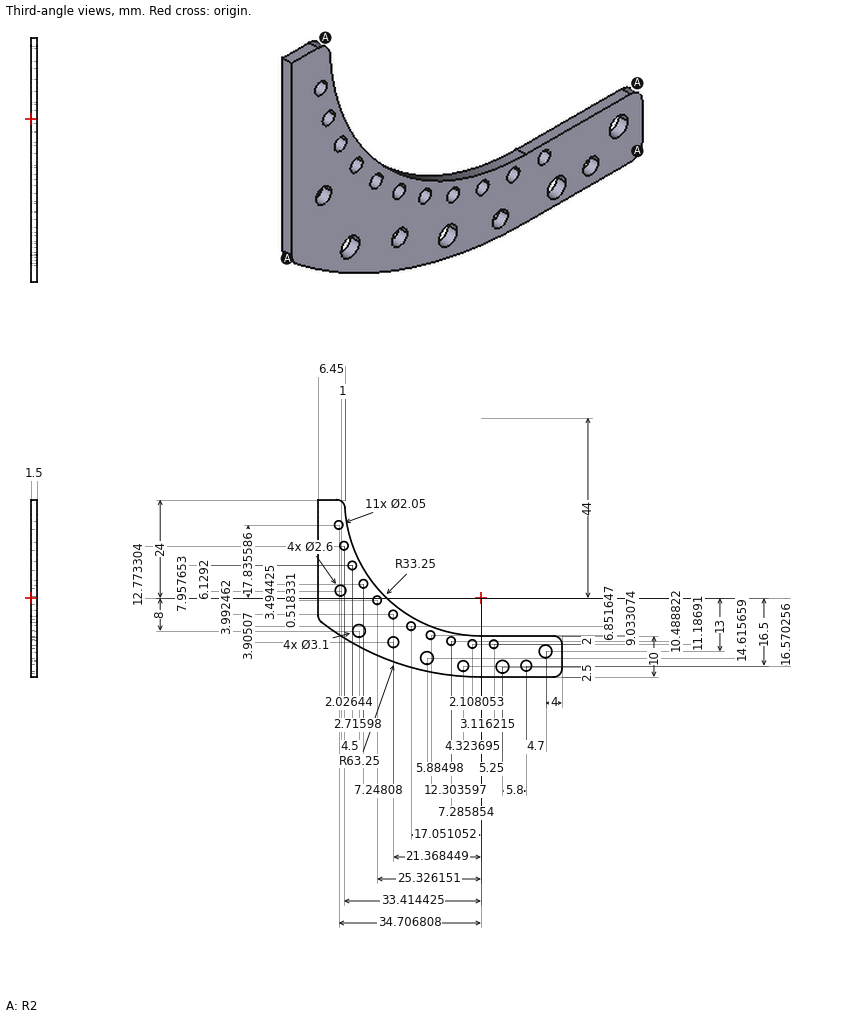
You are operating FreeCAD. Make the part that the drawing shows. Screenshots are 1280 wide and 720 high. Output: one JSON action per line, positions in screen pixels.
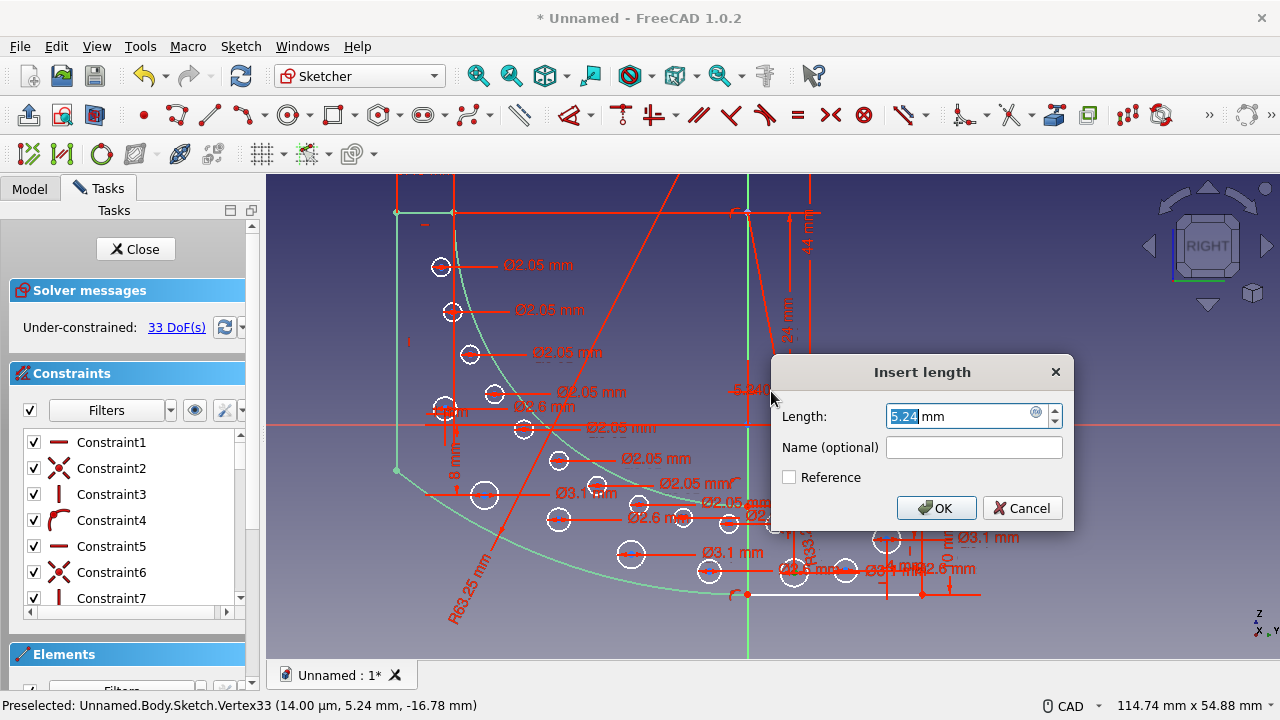
{"action": "type", "text": "5.25"}
{"action": "key", "text": "Return"}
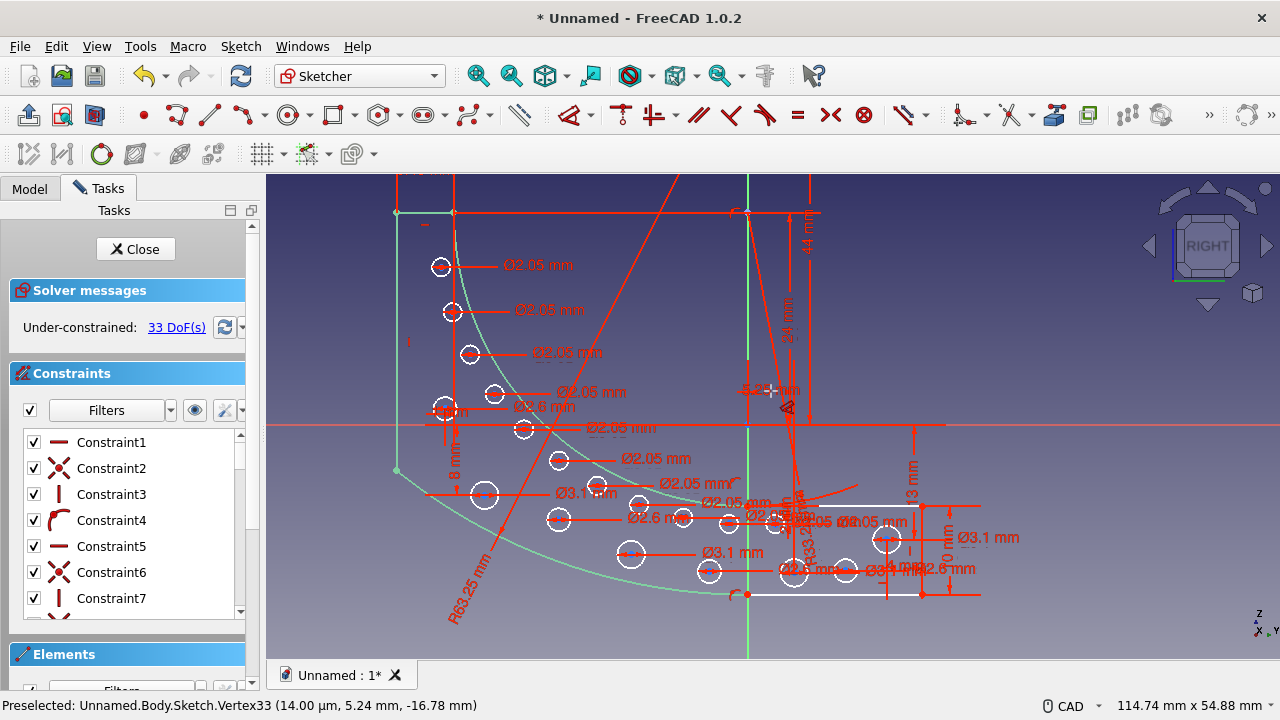
{"action": "left_click", "coordinate": [846, 571]}
{"action": "left_click", "coordinate": [880, 447]}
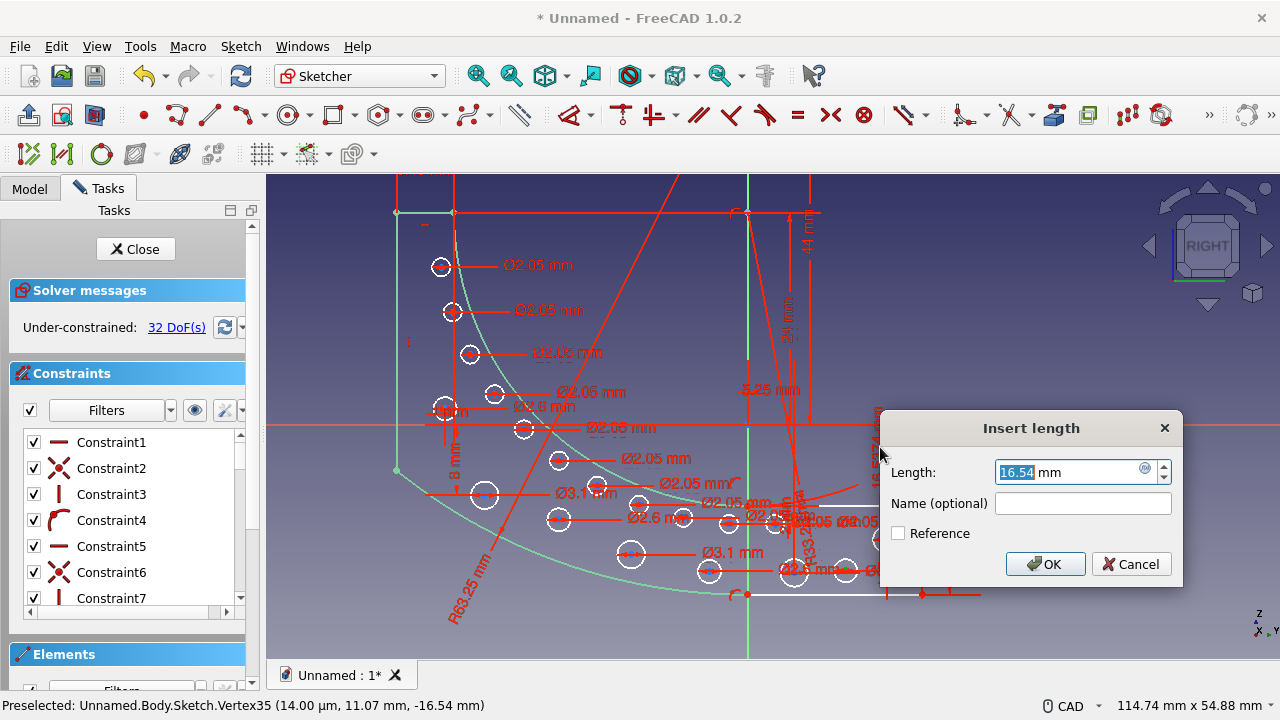
{"action": "type", "text": "16.5"}
{"action": "key", "text": "Return"}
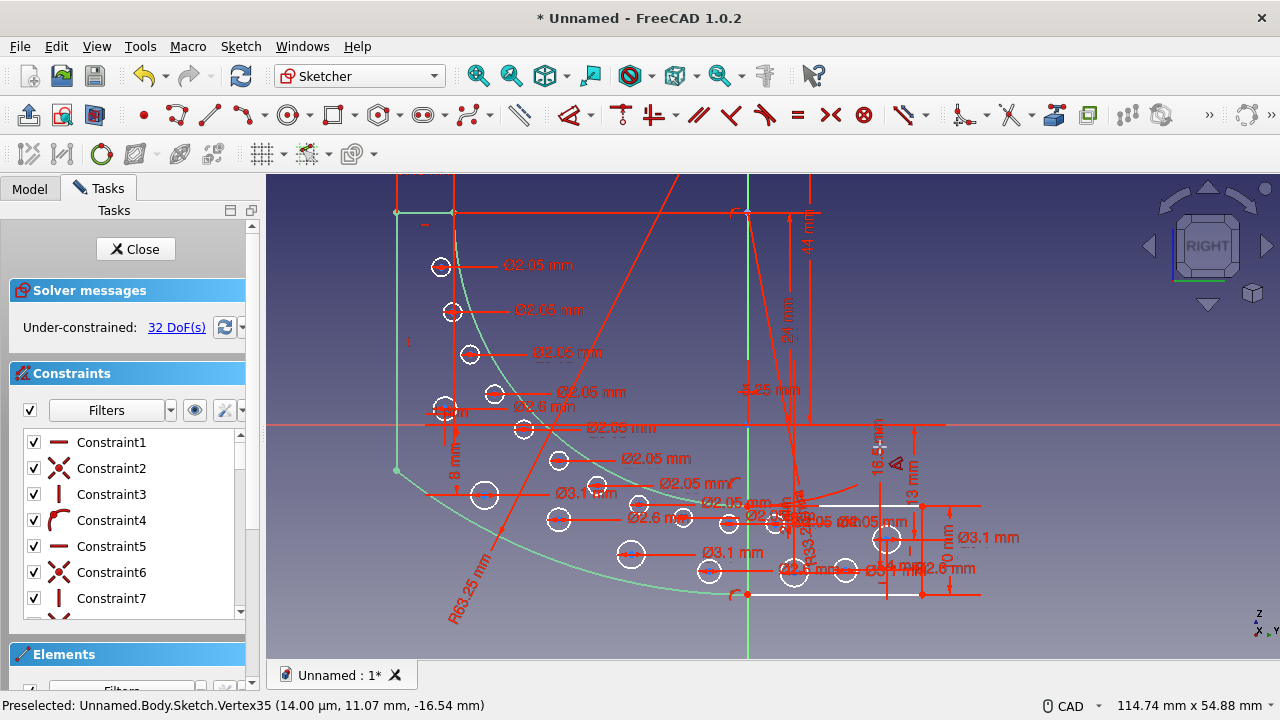
{"action": "left_click", "coordinate": [445, 409]}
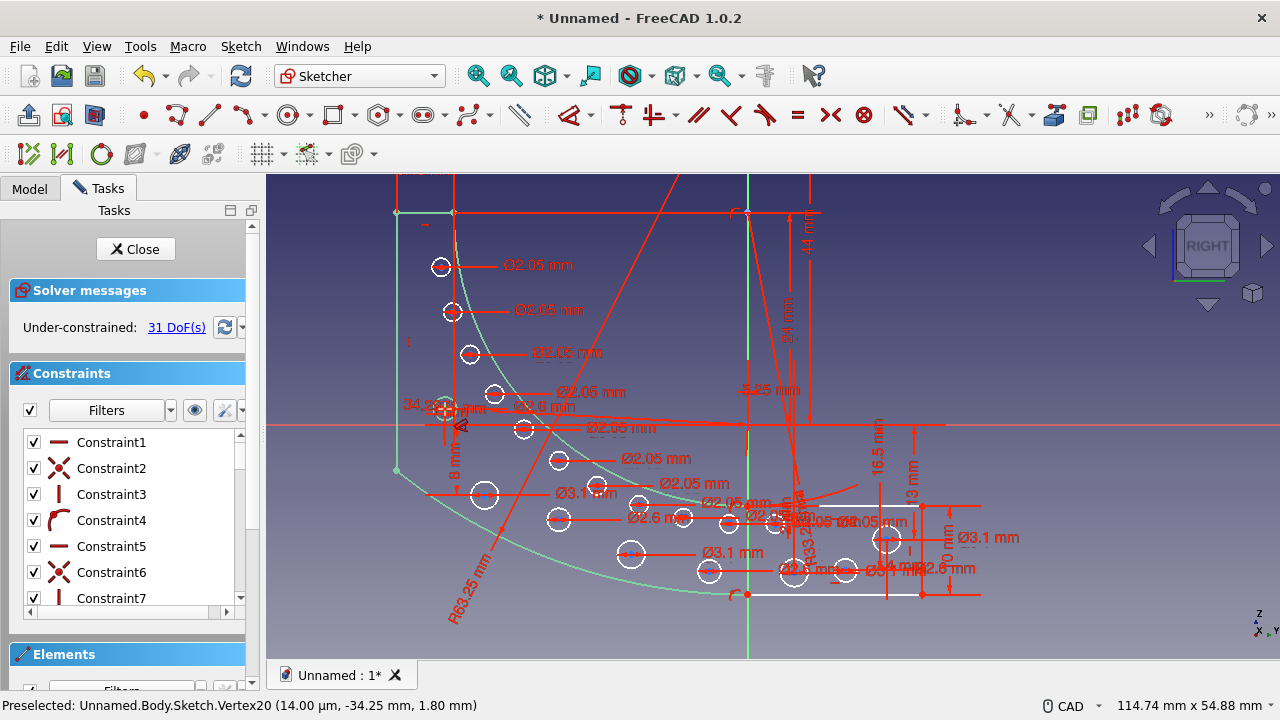
{"action": "left_click", "coordinate": [485, 495]}
{"action": "left_click", "coordinate": [456, 529]}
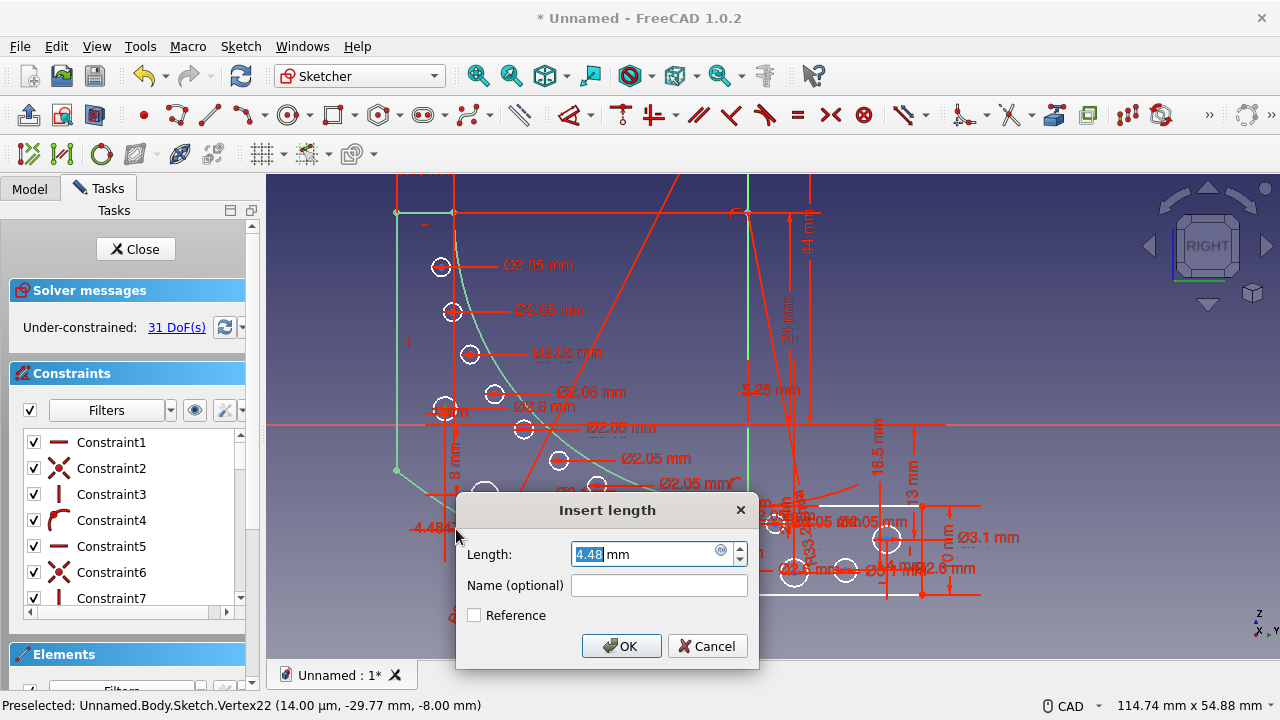
{"action": "type", "text": "4.5"}
{"action": "key", "text": "Return"}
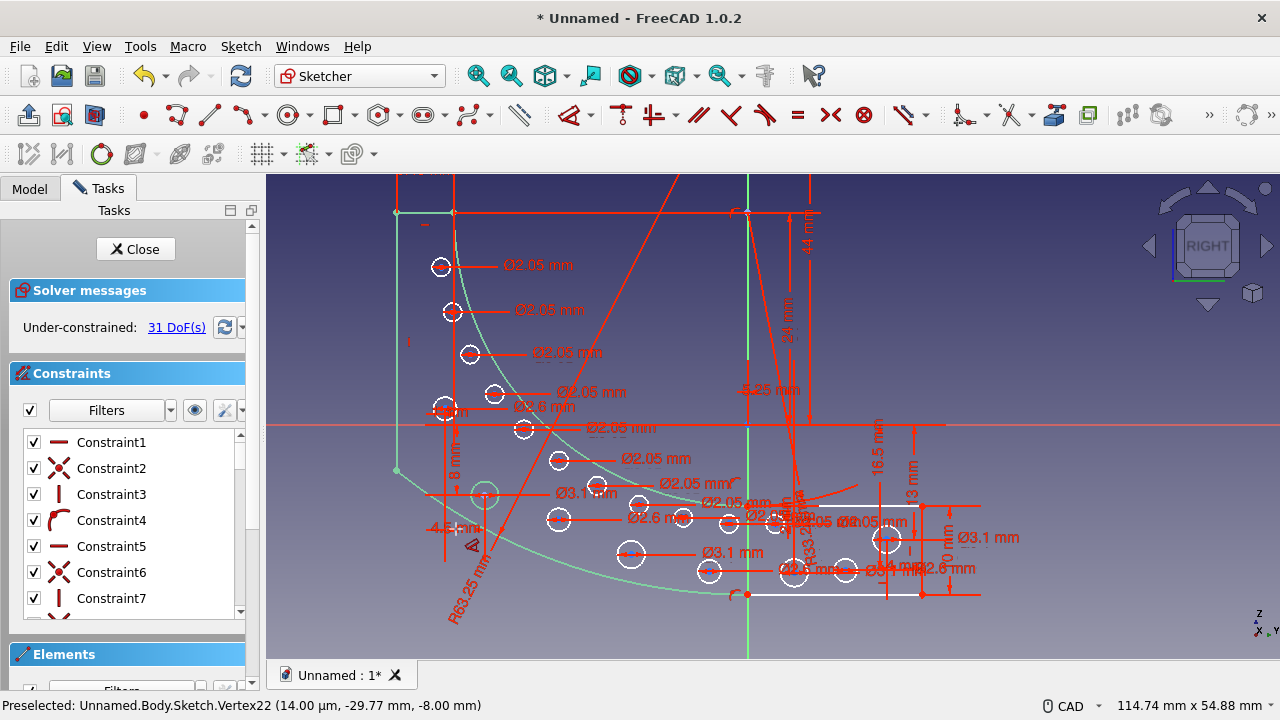
{"action": "scroll", "coordinate": [748, 595], "scroll_direction": "up", "scroll_amount": 3}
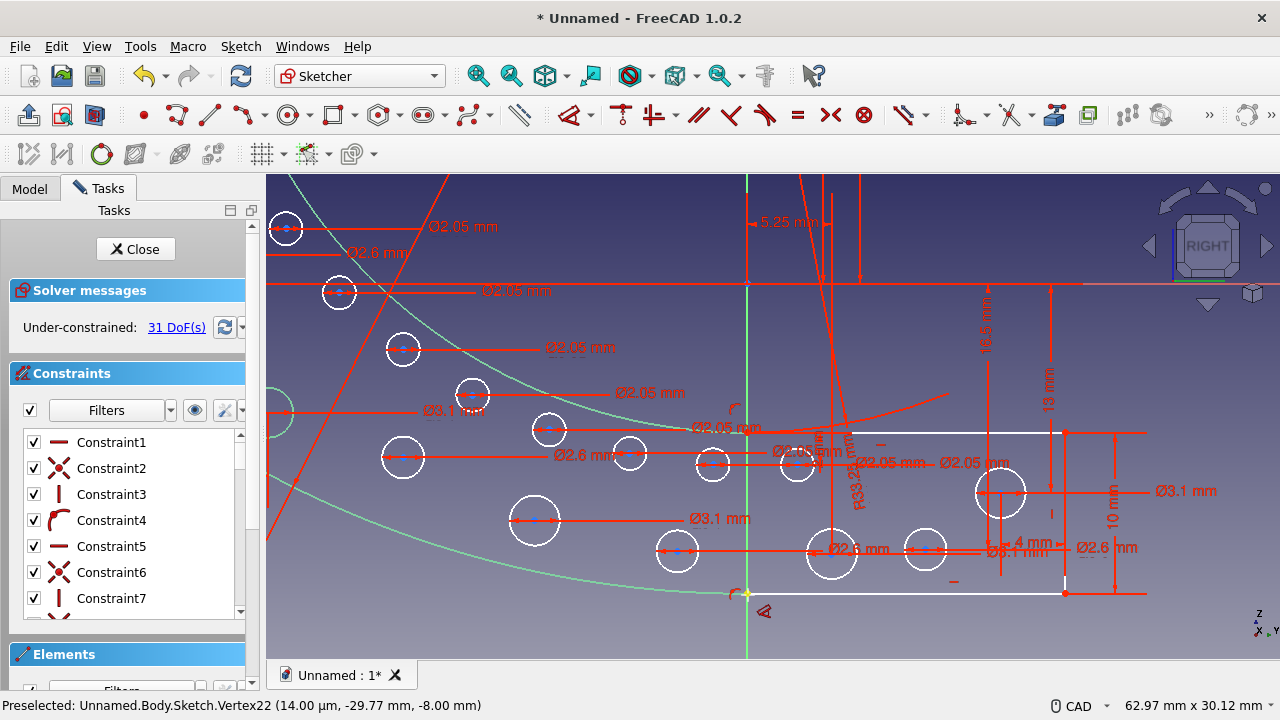
{"action": "left_click", "coordinate": [747, 594]}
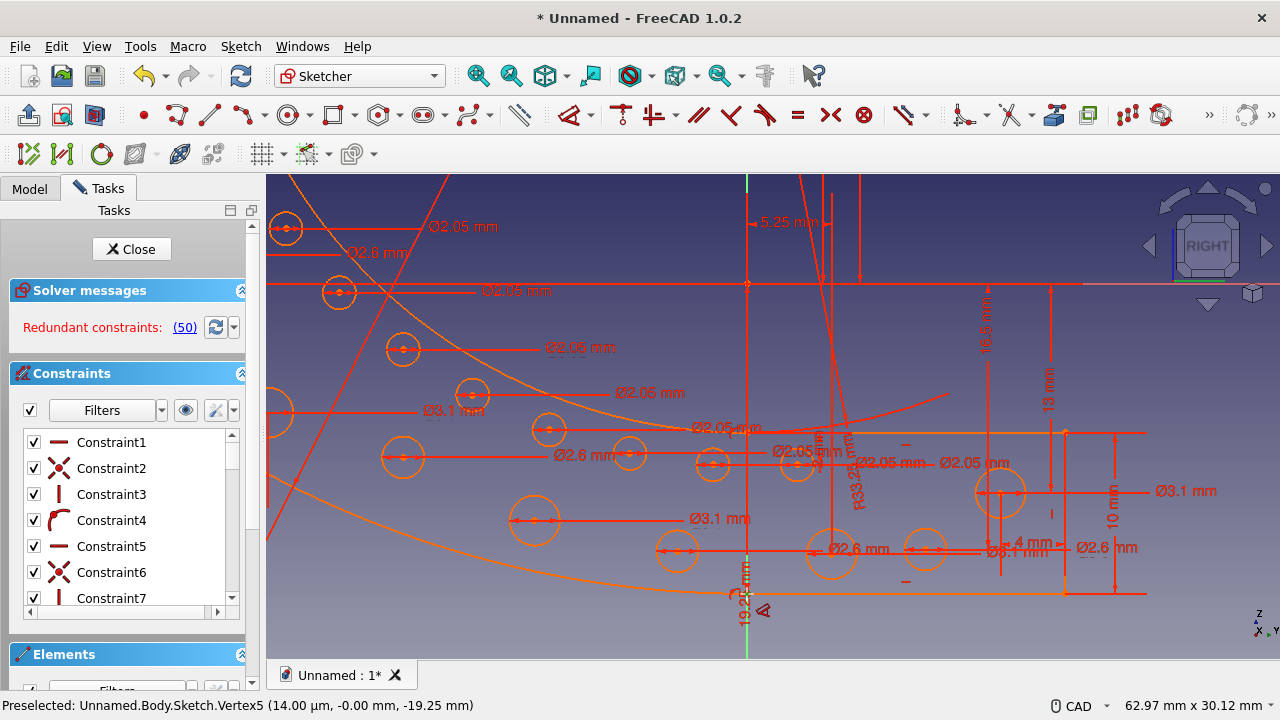
{"action": "left_click", "coordinate": [832, 554]}
{"action": "left_click", "coordinate": [866, 574]}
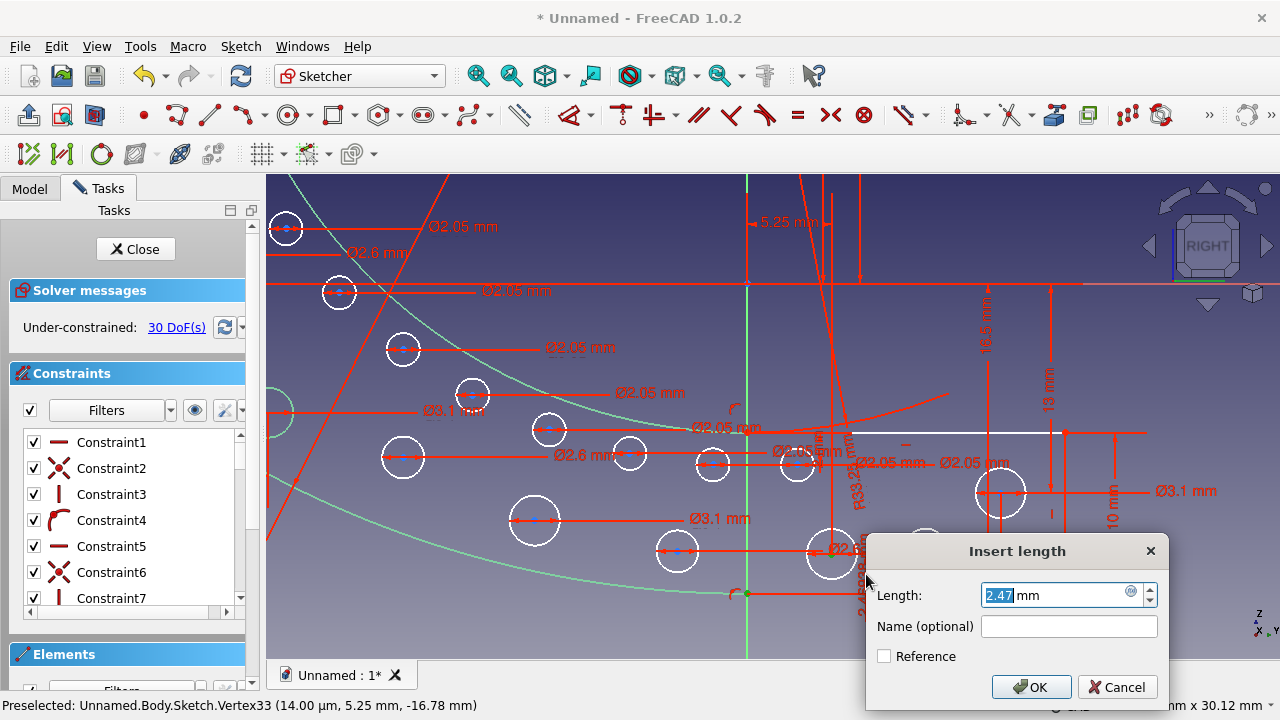
{"action": "type", "text": "2.5"}
{"action": "key", "text": "Return"}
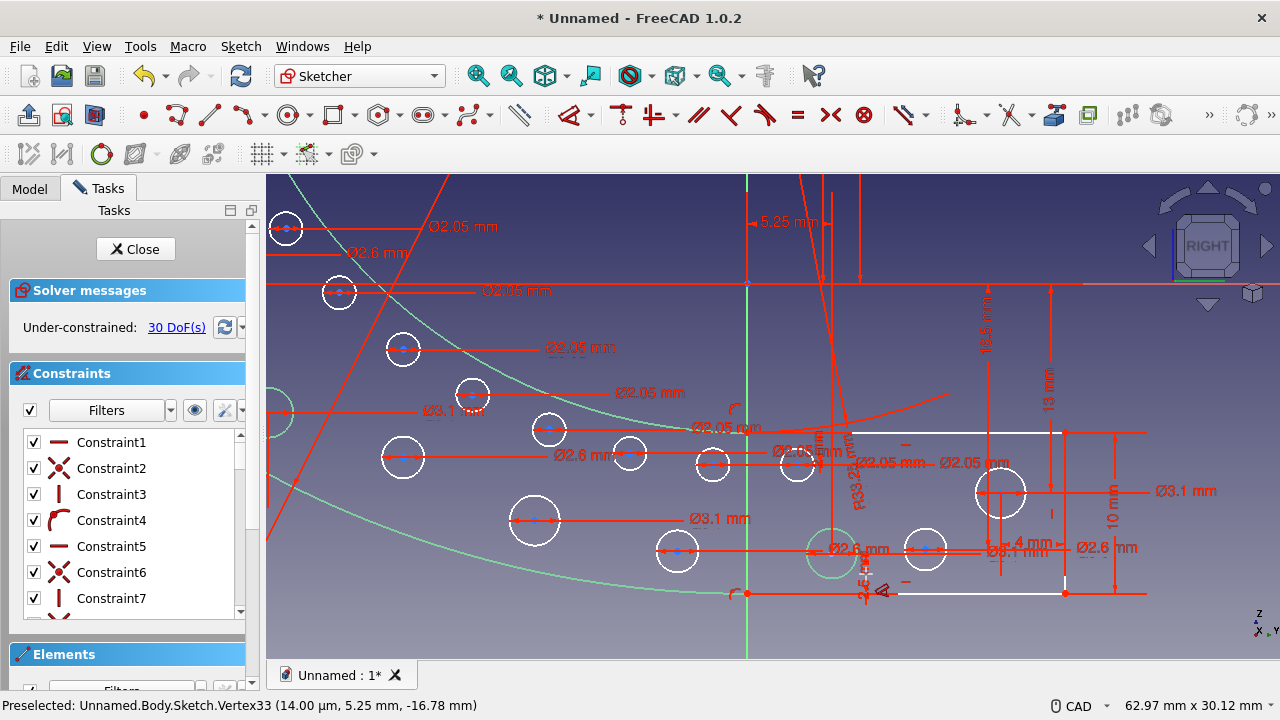
{"action": "left_click", "coordinate": [832, 554]}